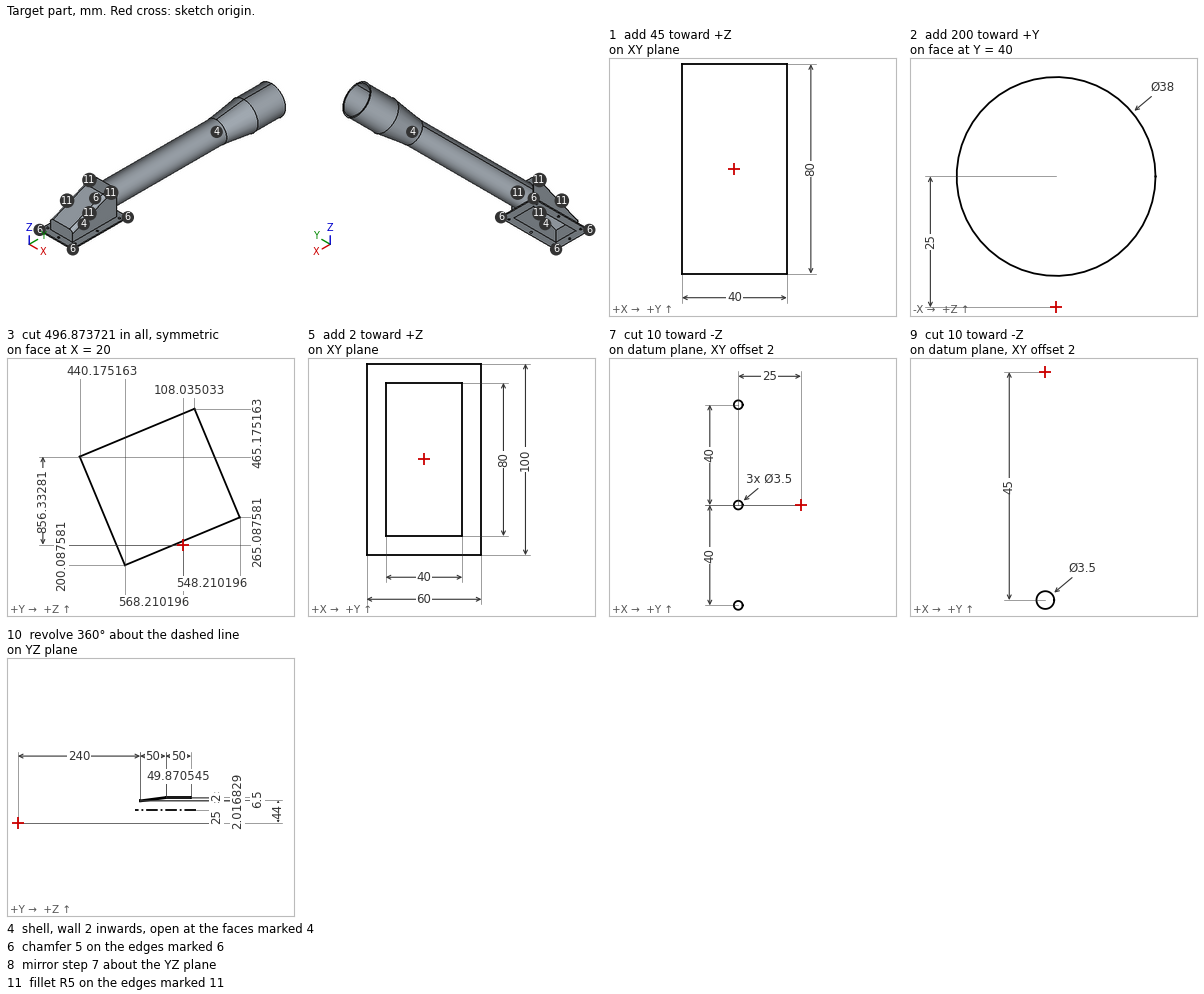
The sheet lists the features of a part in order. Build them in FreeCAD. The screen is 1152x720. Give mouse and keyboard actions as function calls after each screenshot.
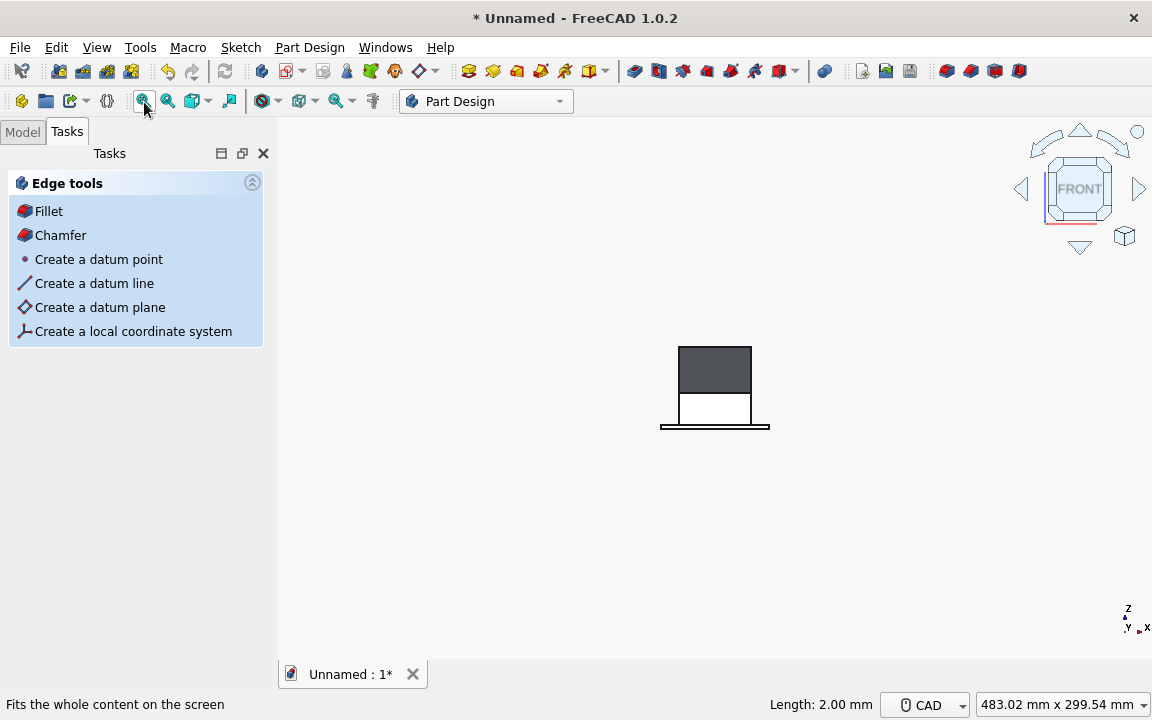
click(144, 102)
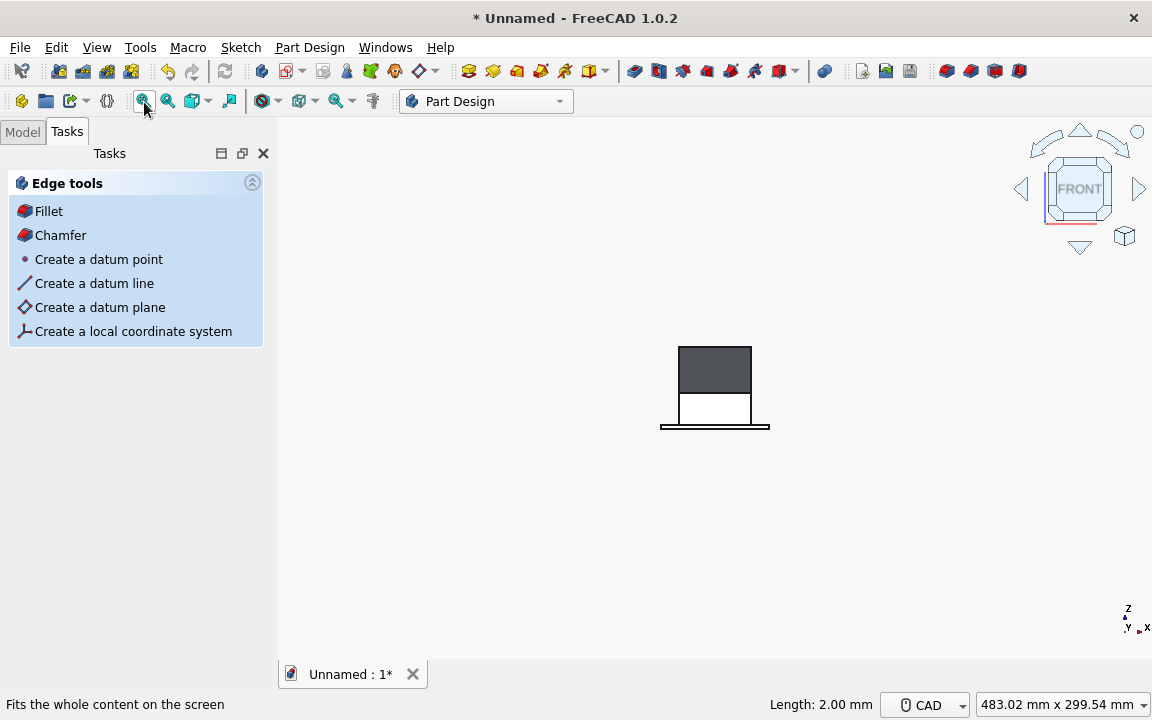
scroll(661, 426, up, 13)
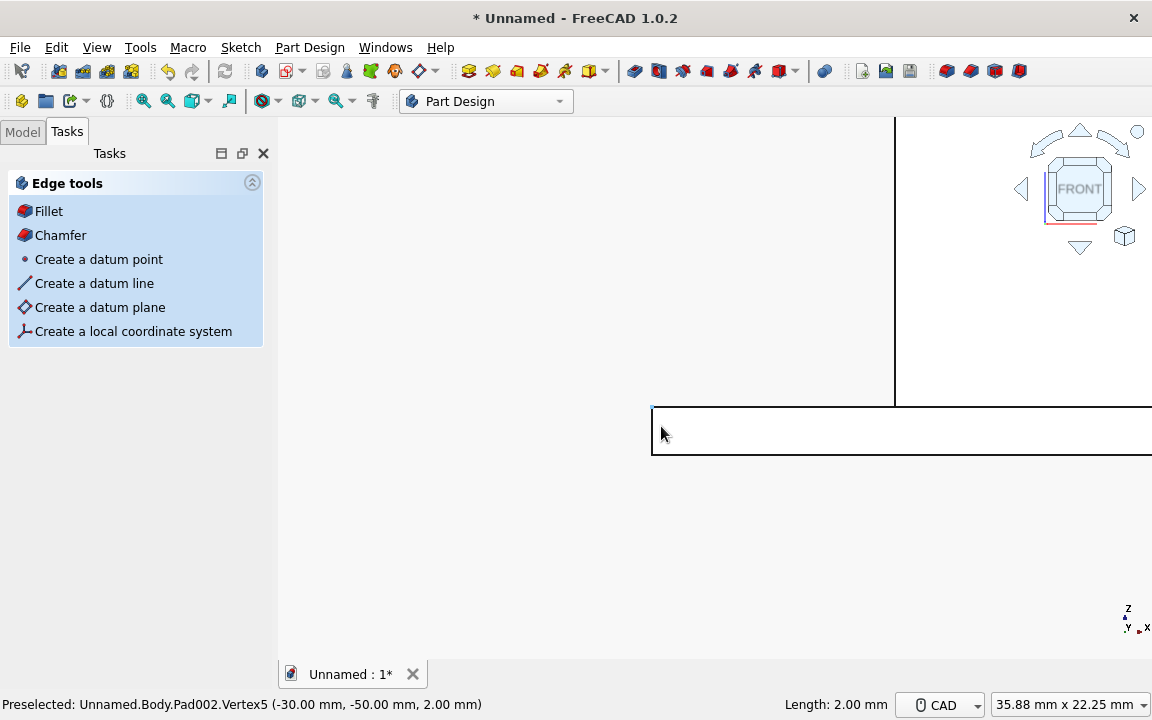
click(652, 430, ctrl)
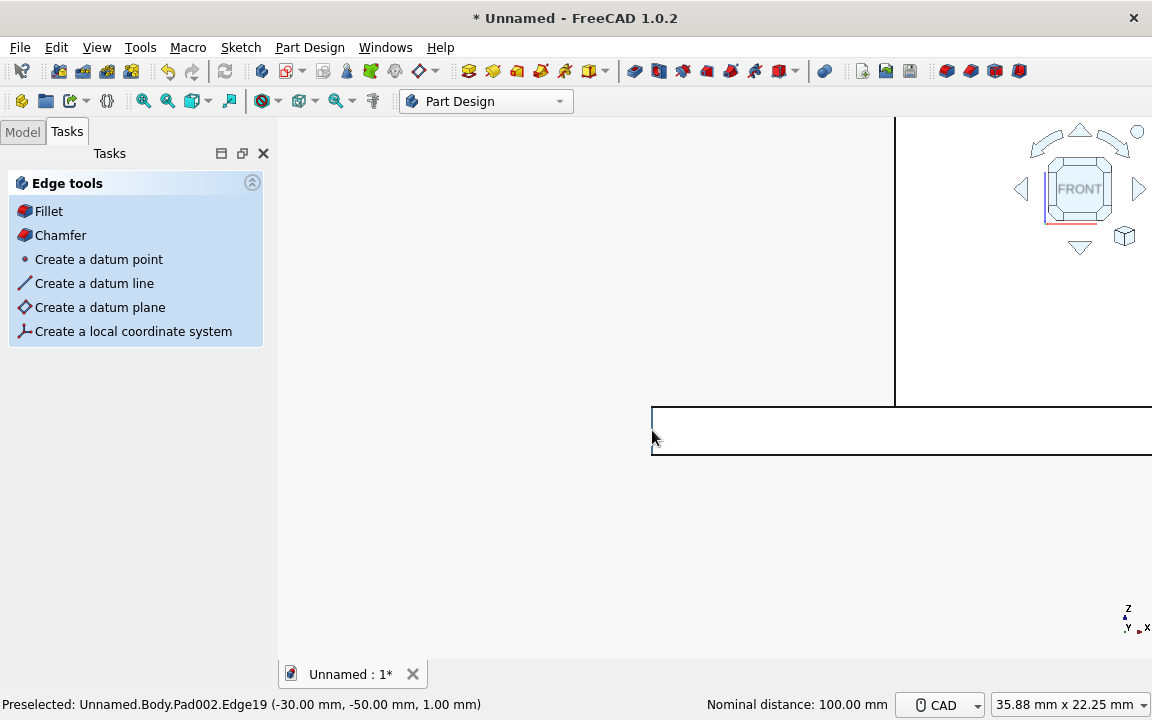
click(144, 102)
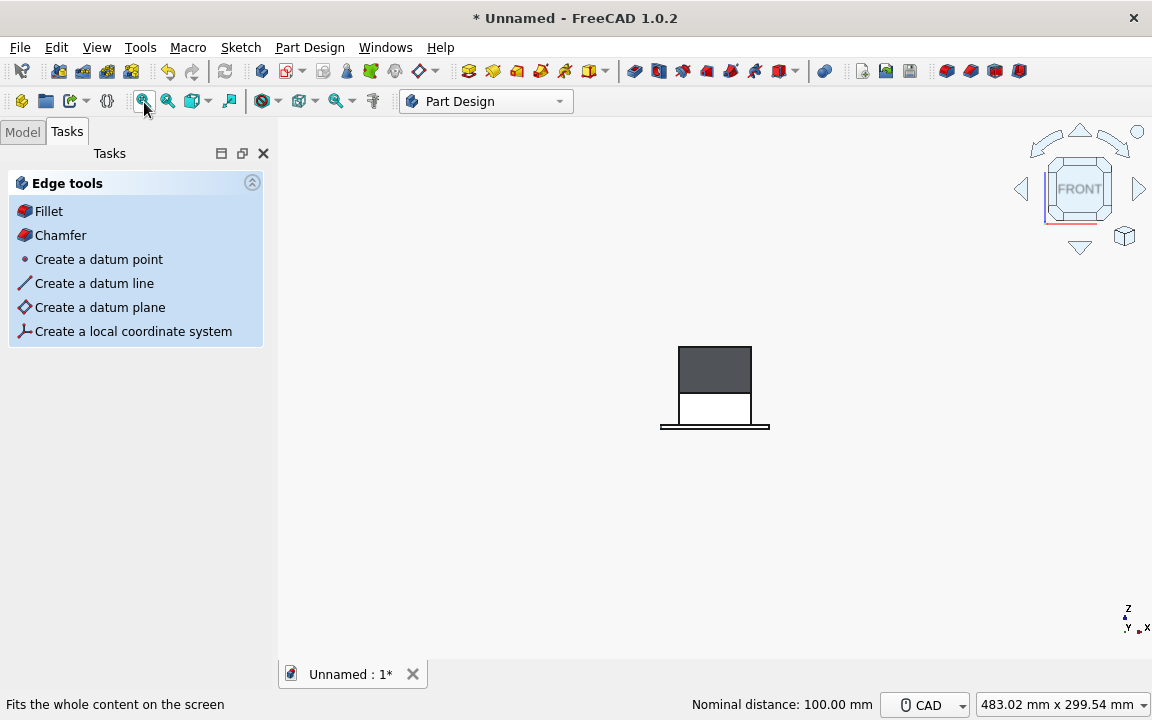
key(3)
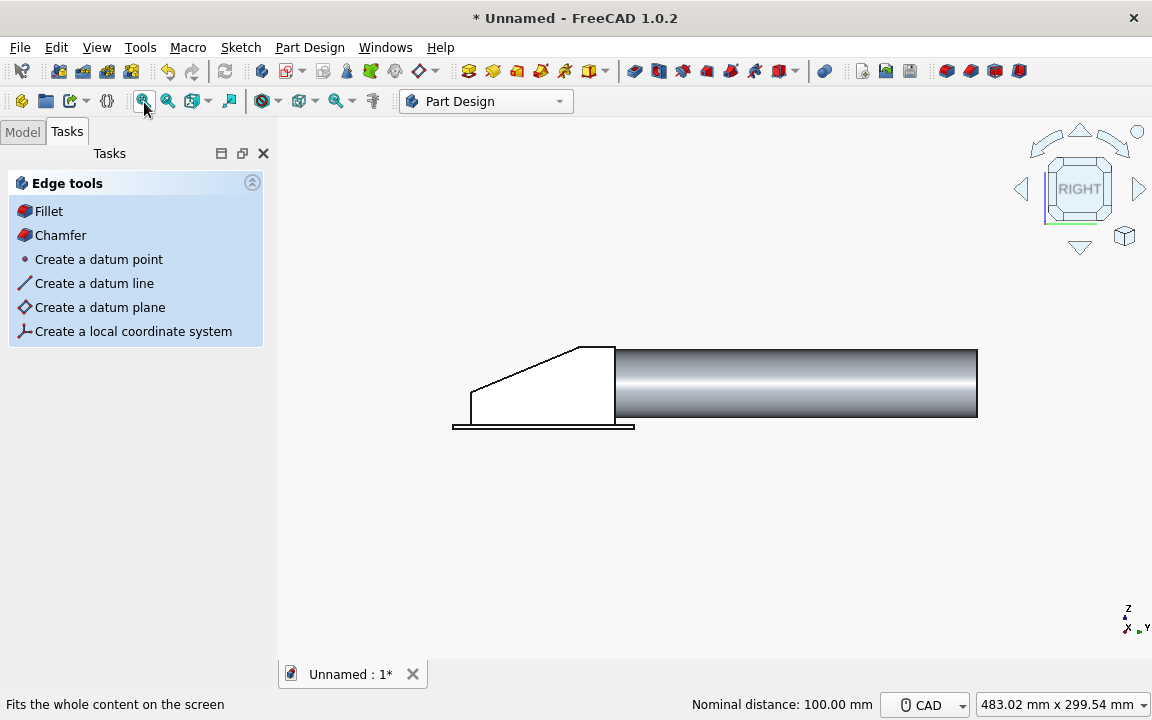
scroll(453, 426, up, 13)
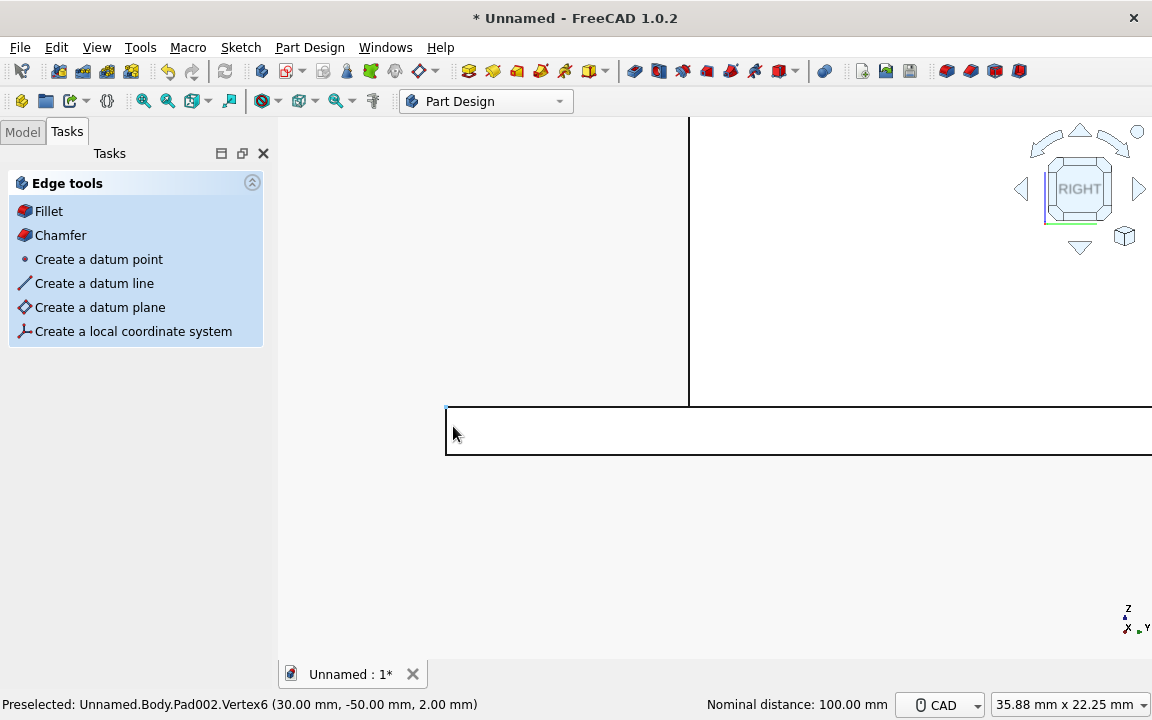
click(446, 430, ctrl)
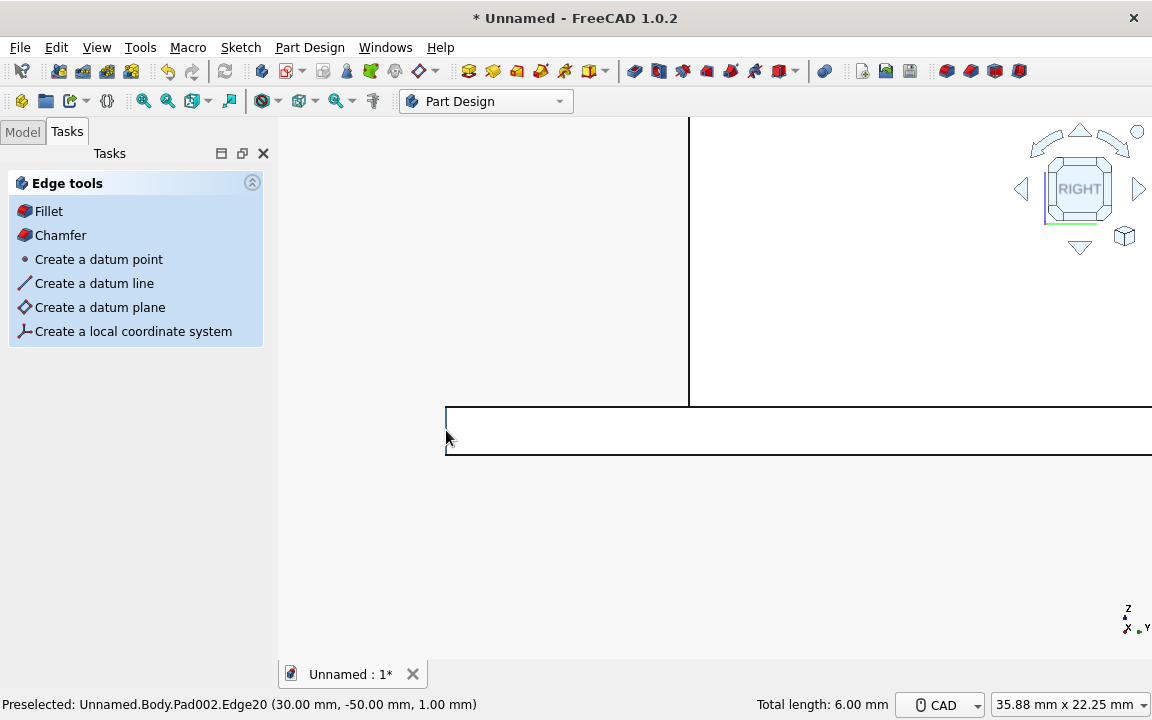
click(144, 102)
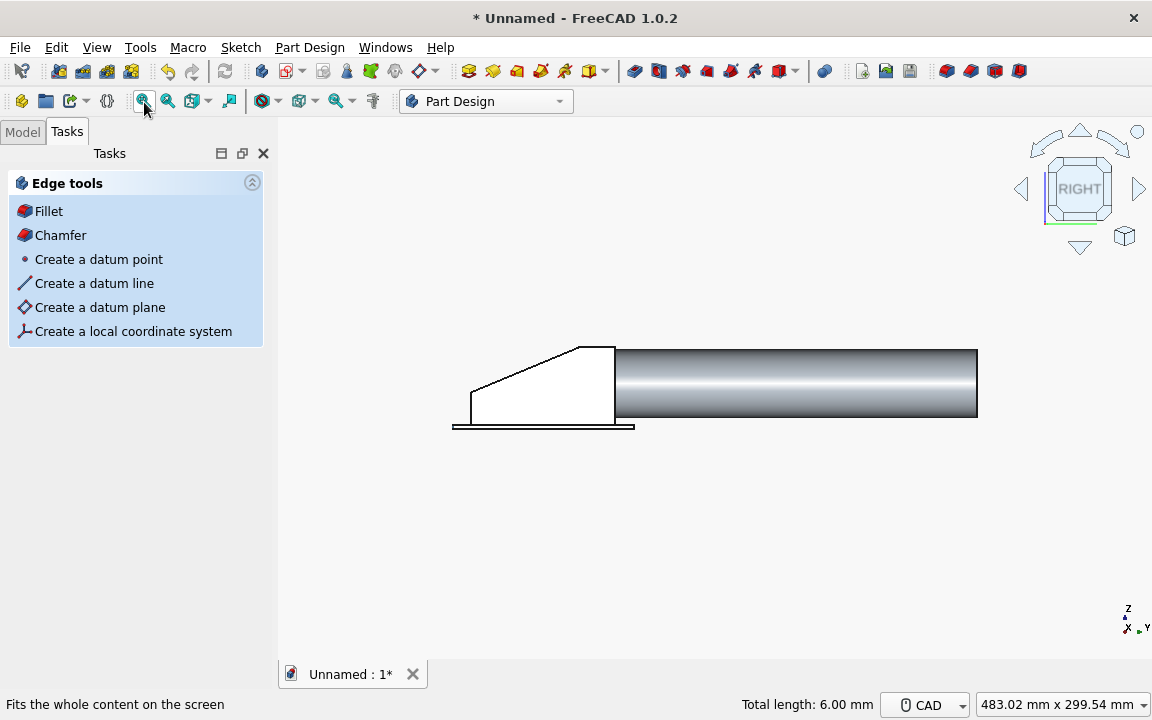
key(5)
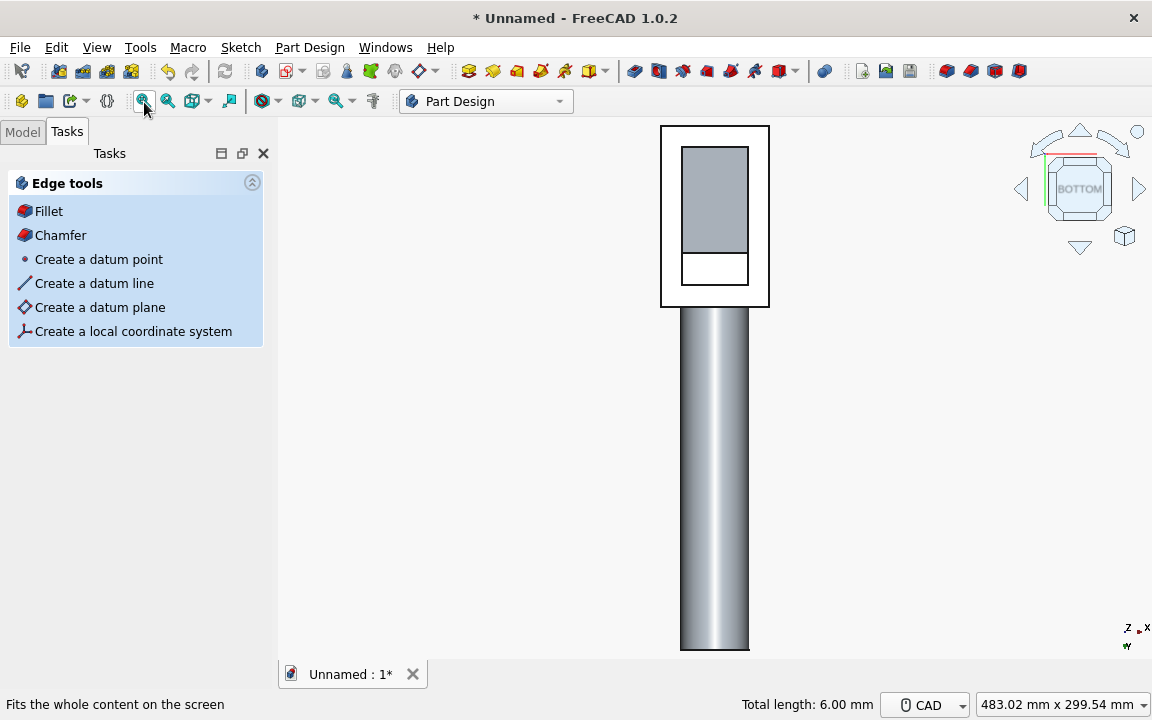
scroll(769, 306, up, 13)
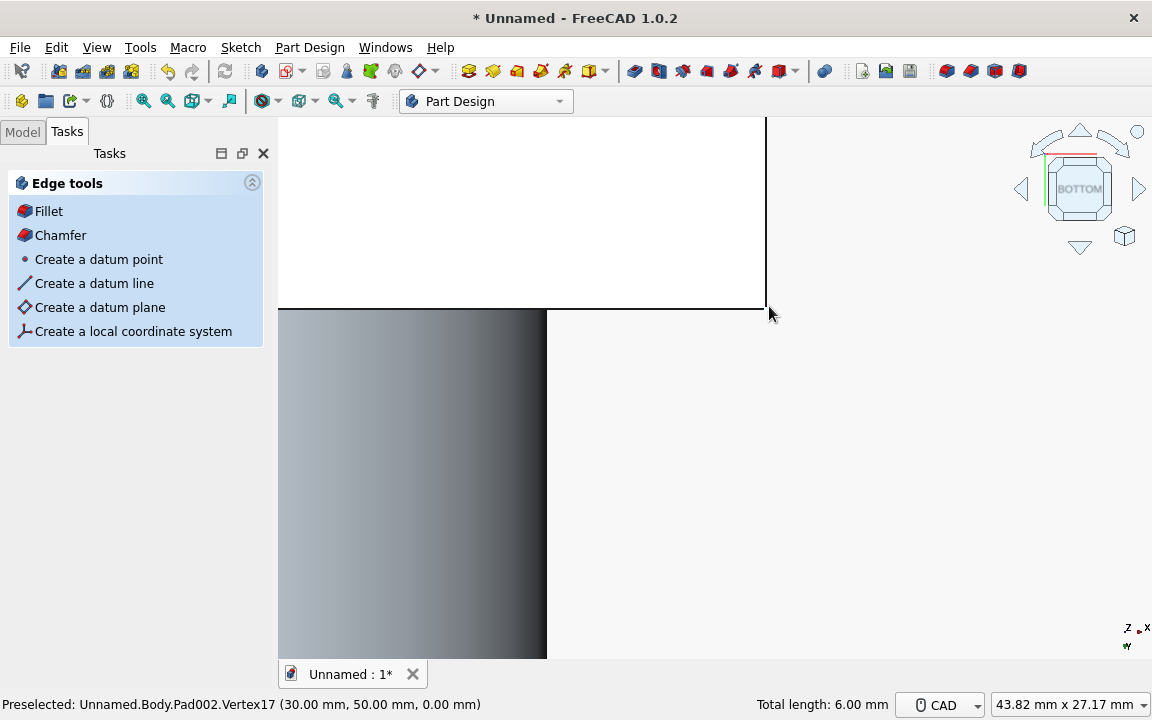
click(144, 102)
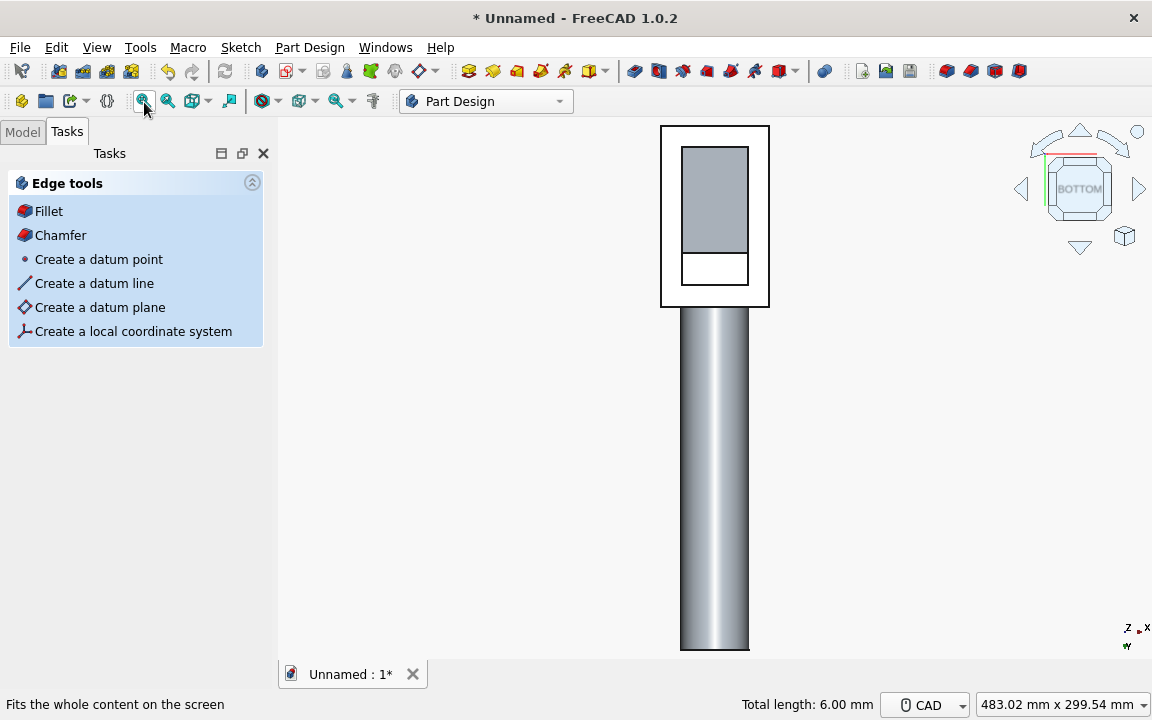
key(4)